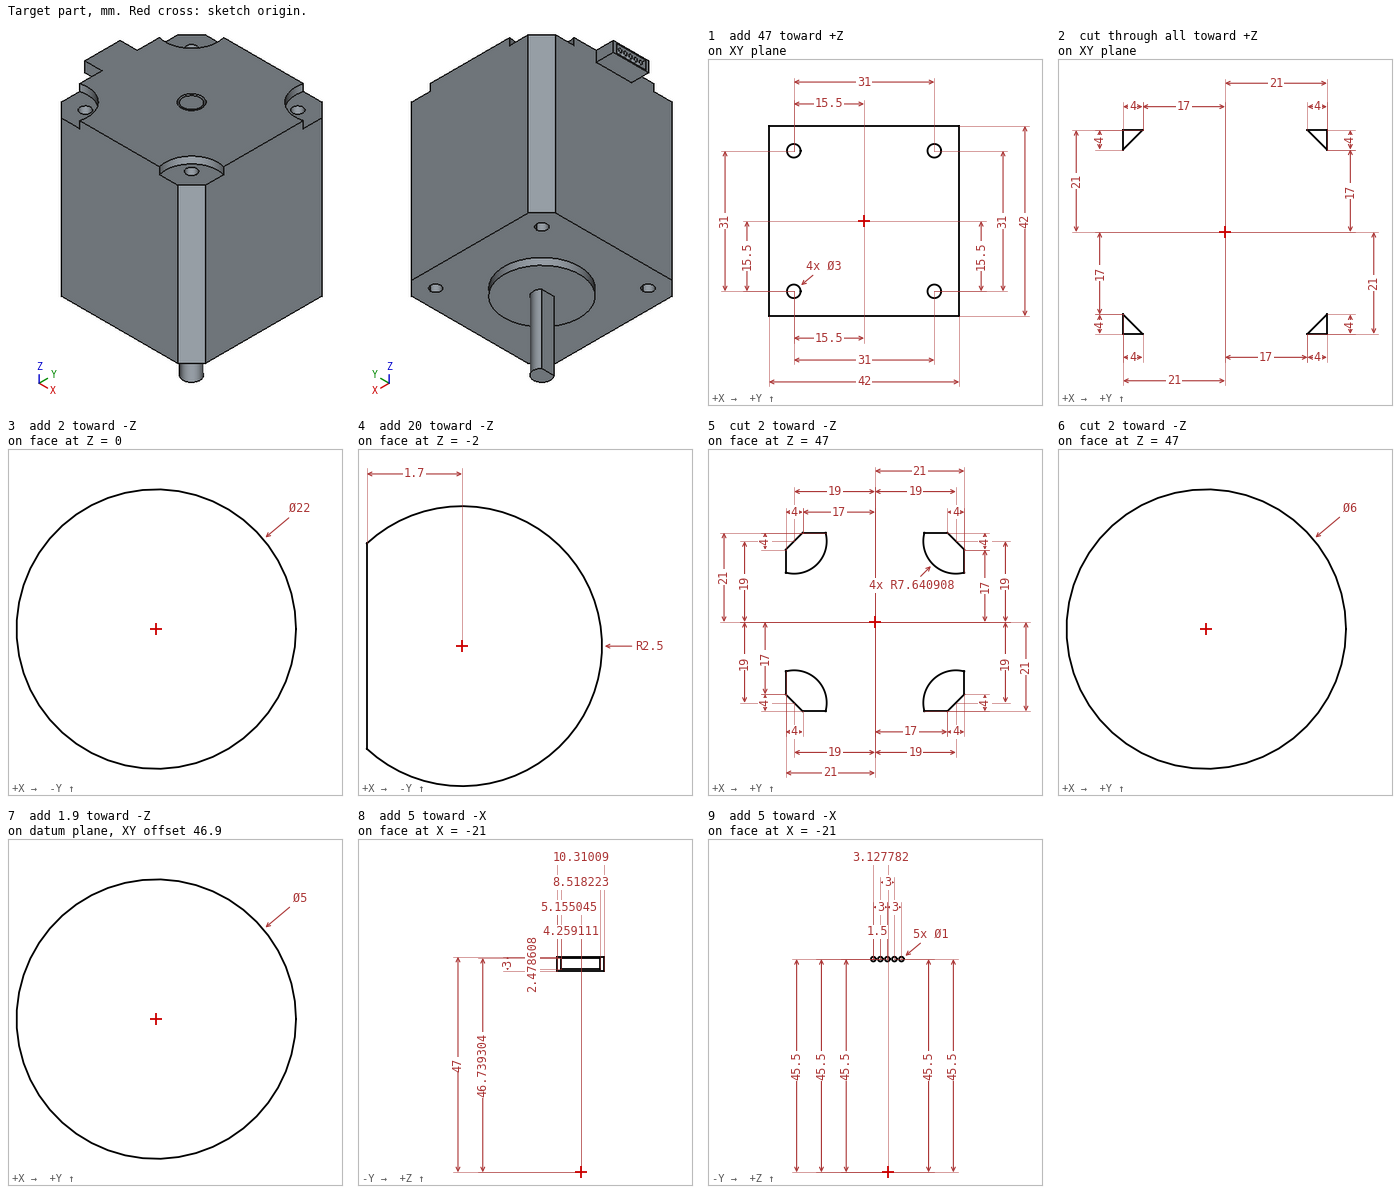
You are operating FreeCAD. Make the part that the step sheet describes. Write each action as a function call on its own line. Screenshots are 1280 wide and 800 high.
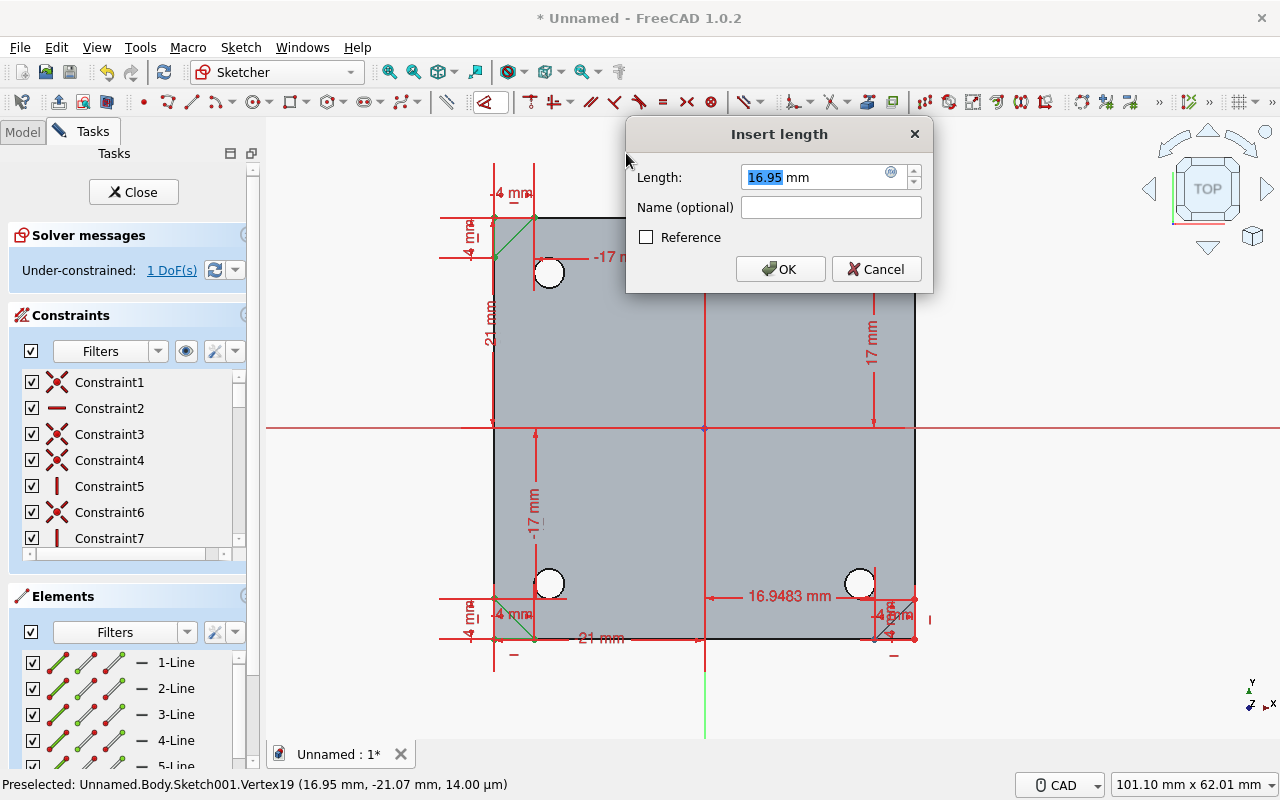
text(17)
key(Return)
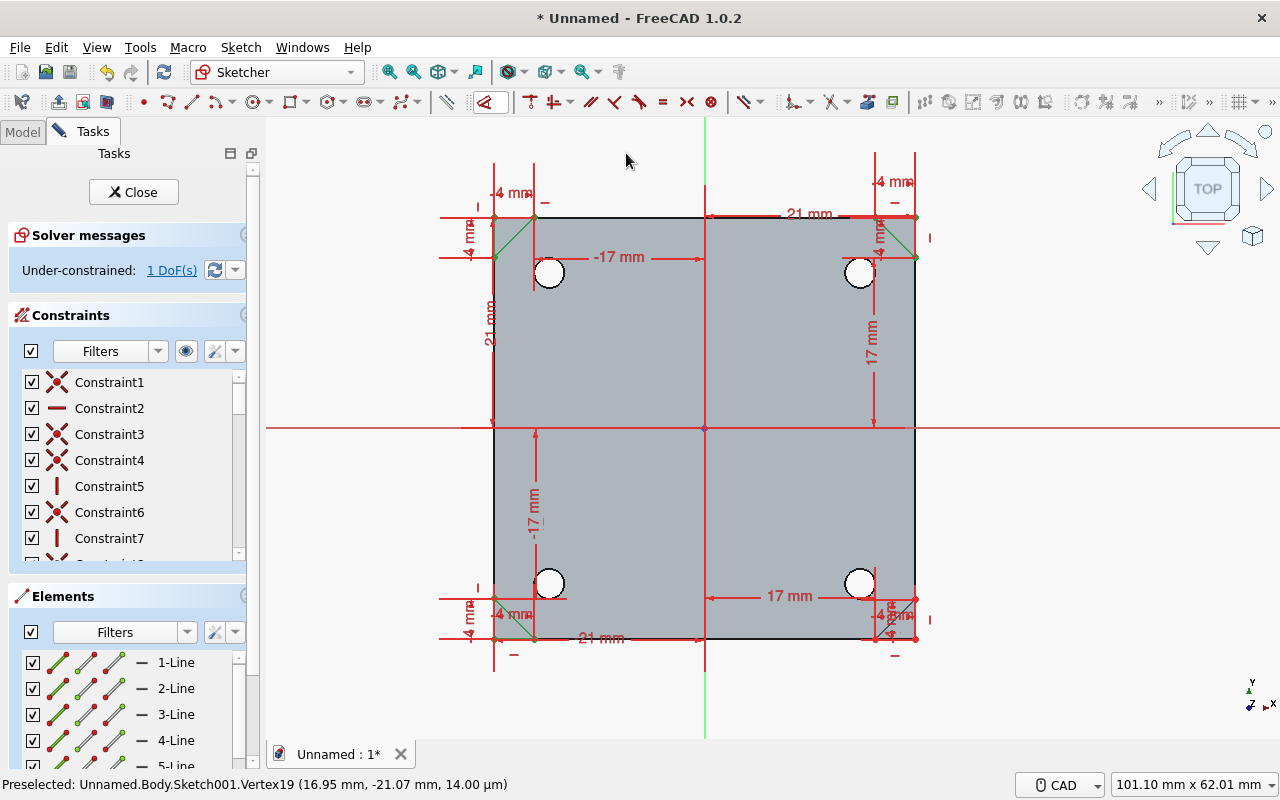
click(875, 640)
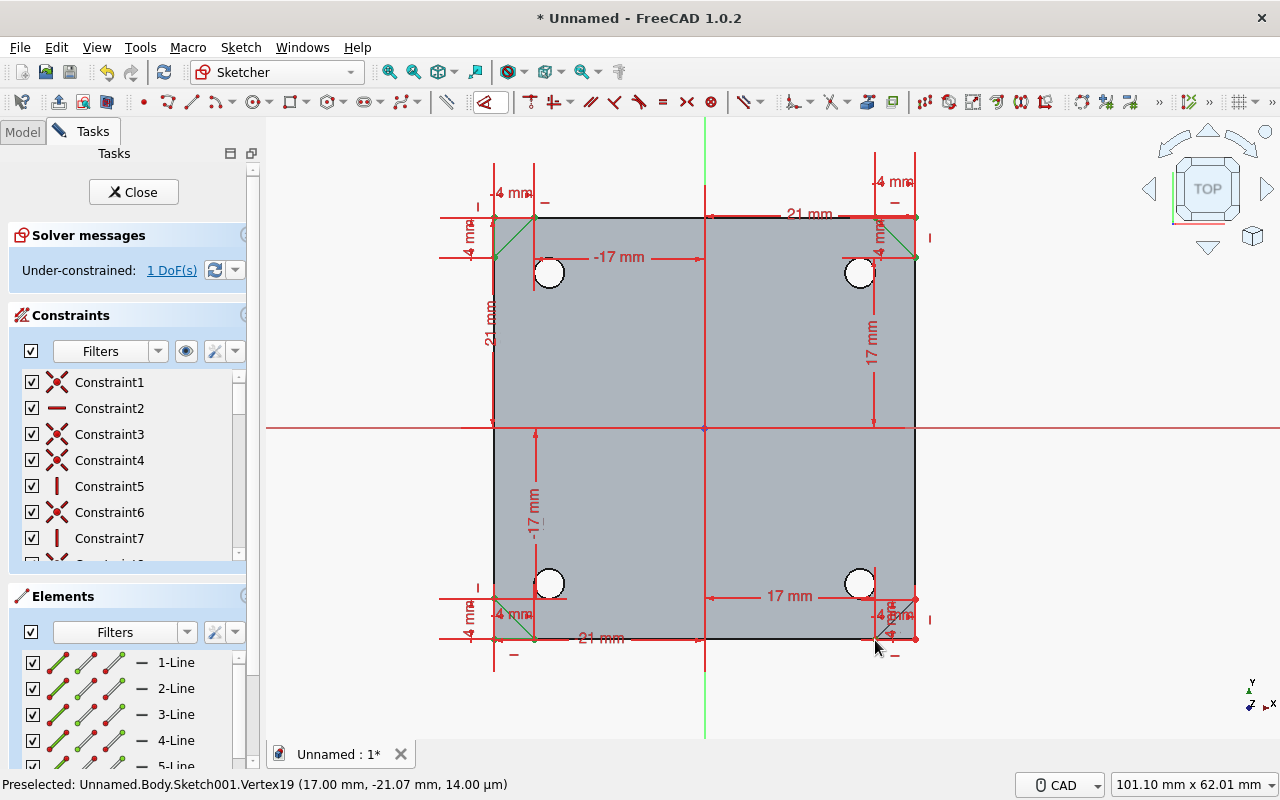
key(i)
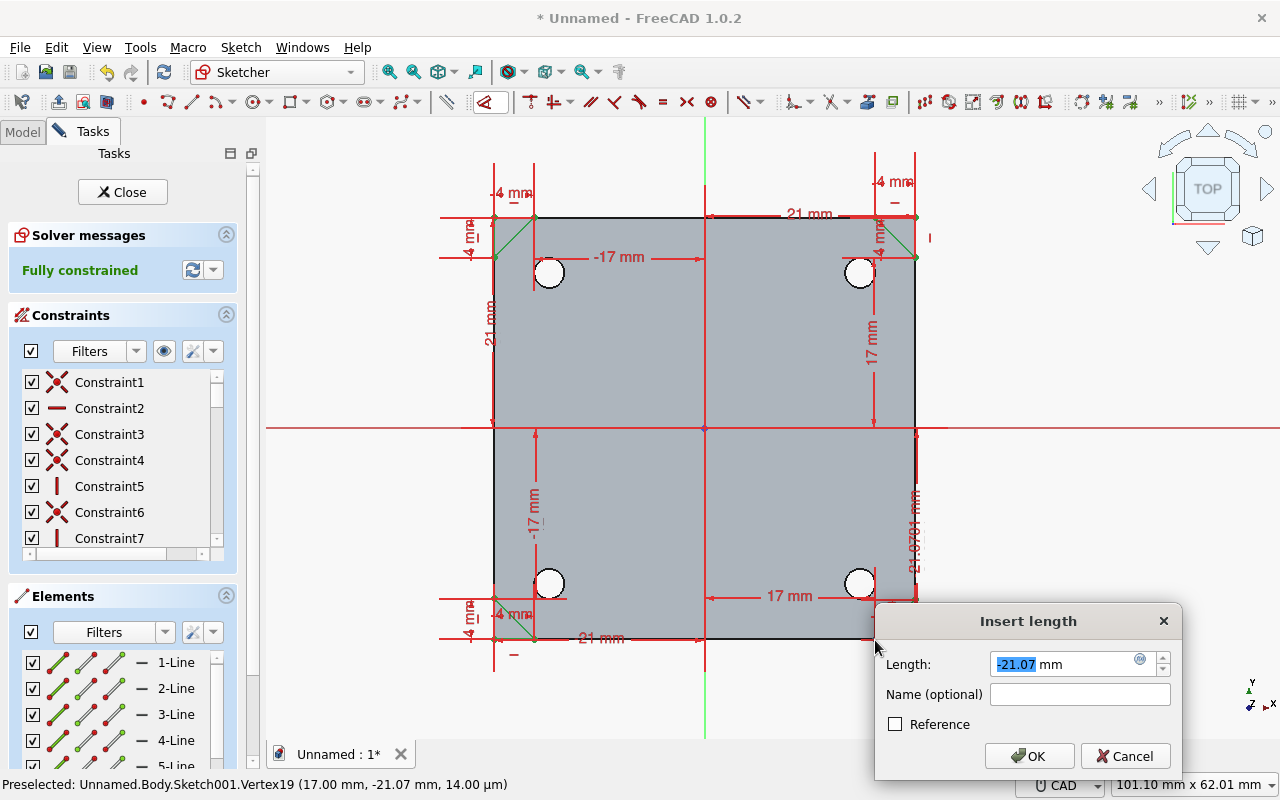
text(-21)
key(Return)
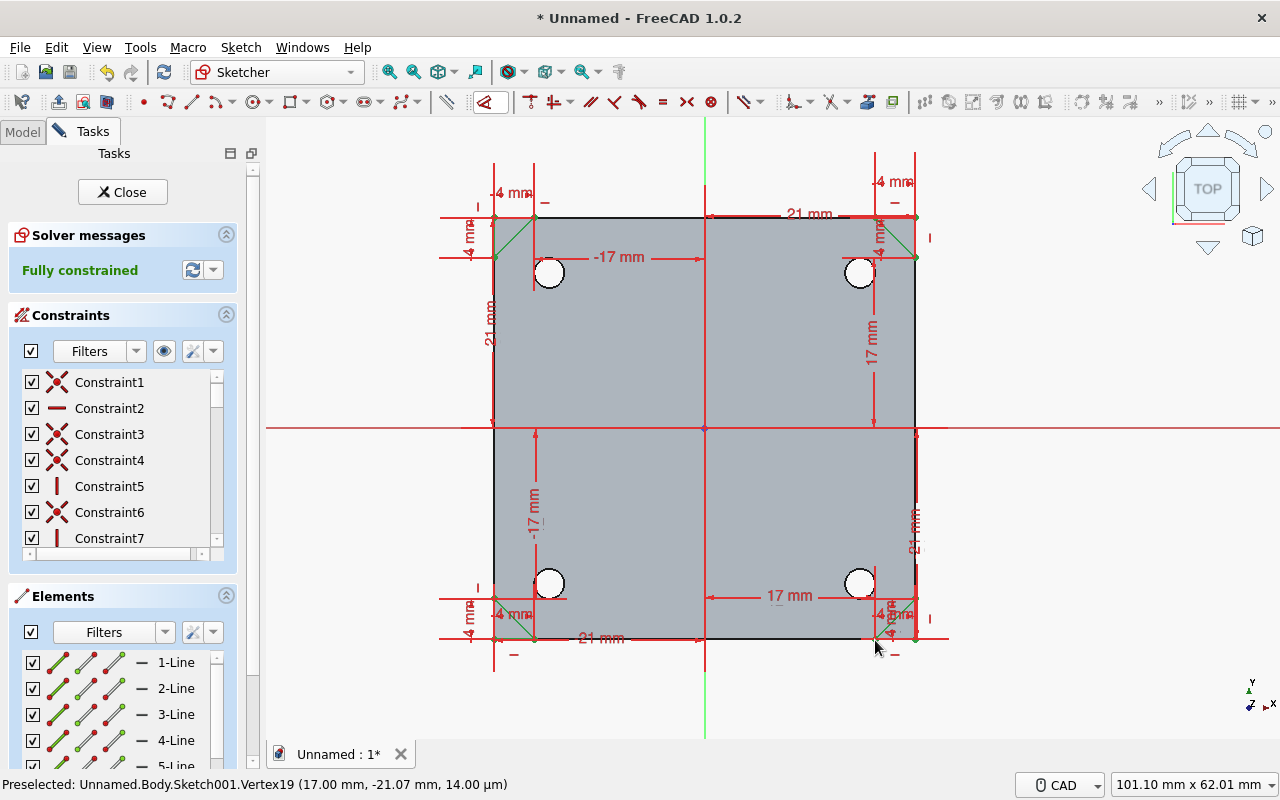
click(123, 192)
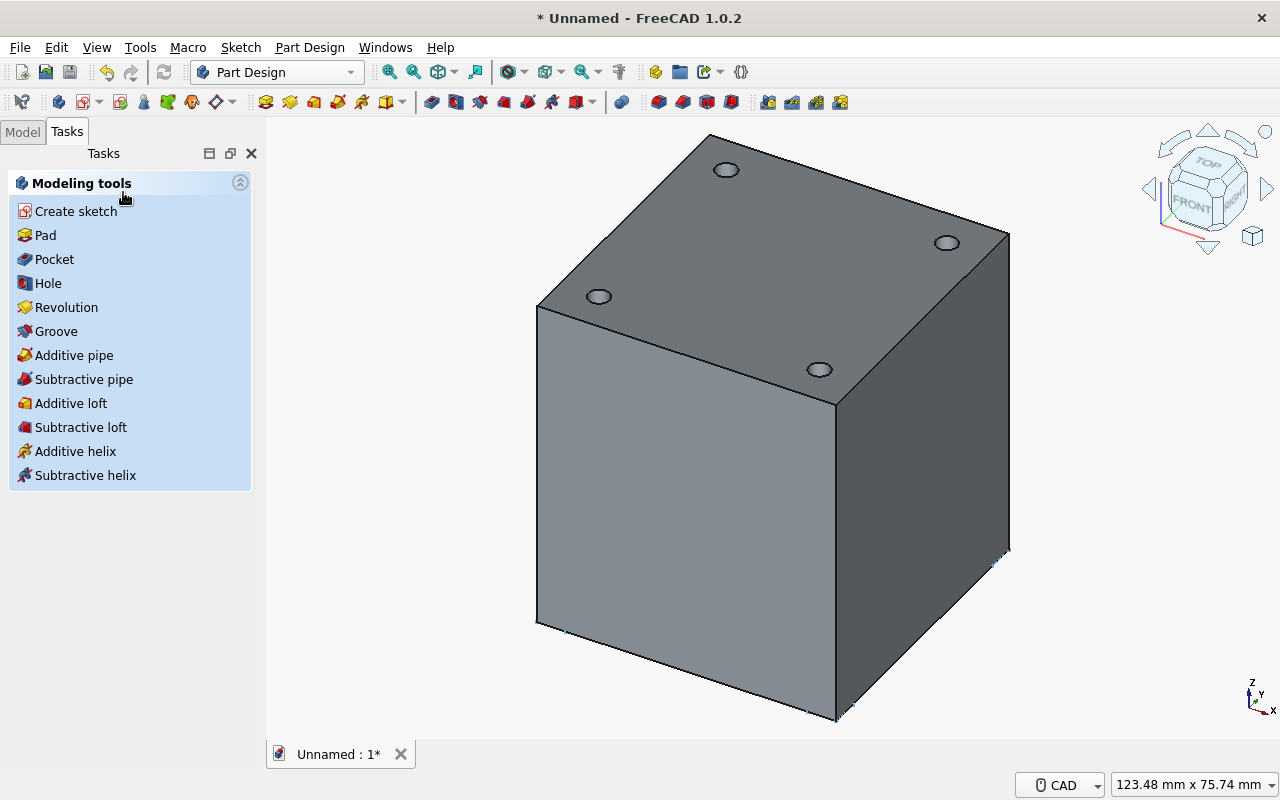
click(432, 102)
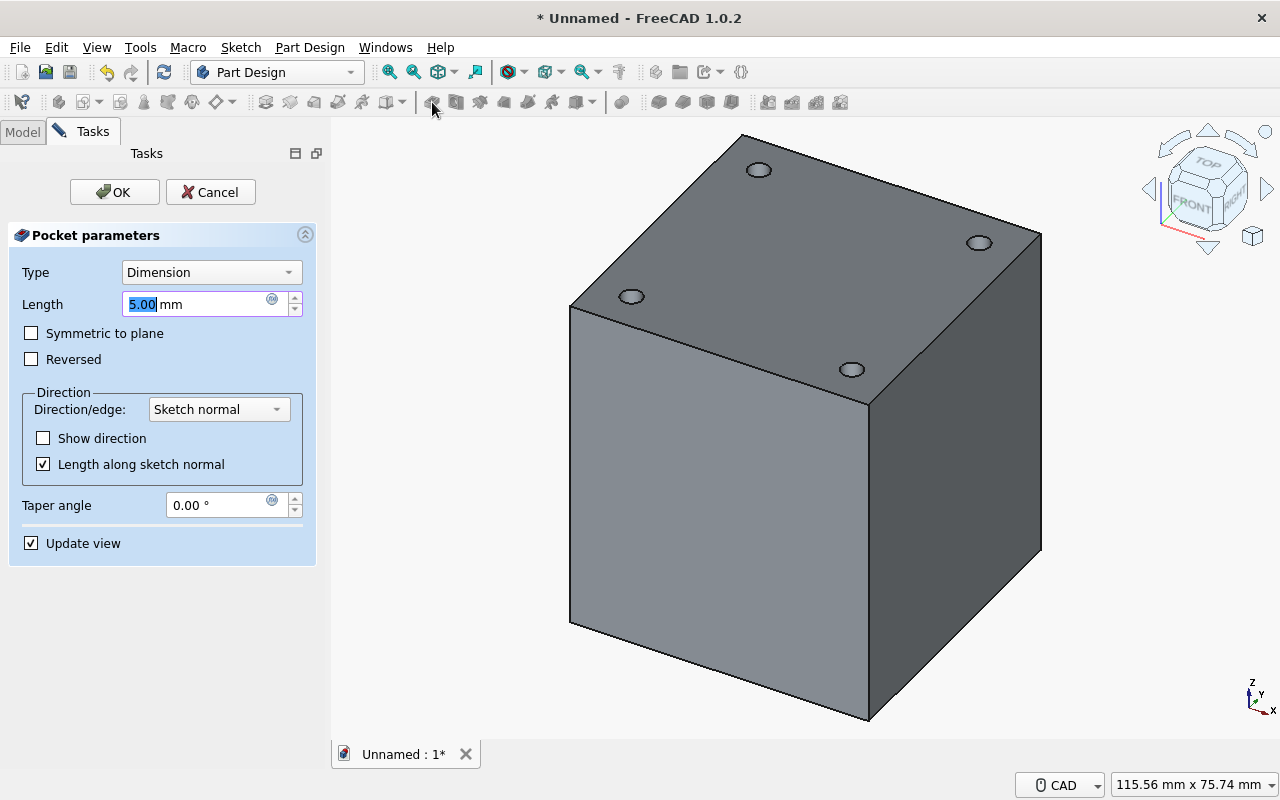
click(212, 272)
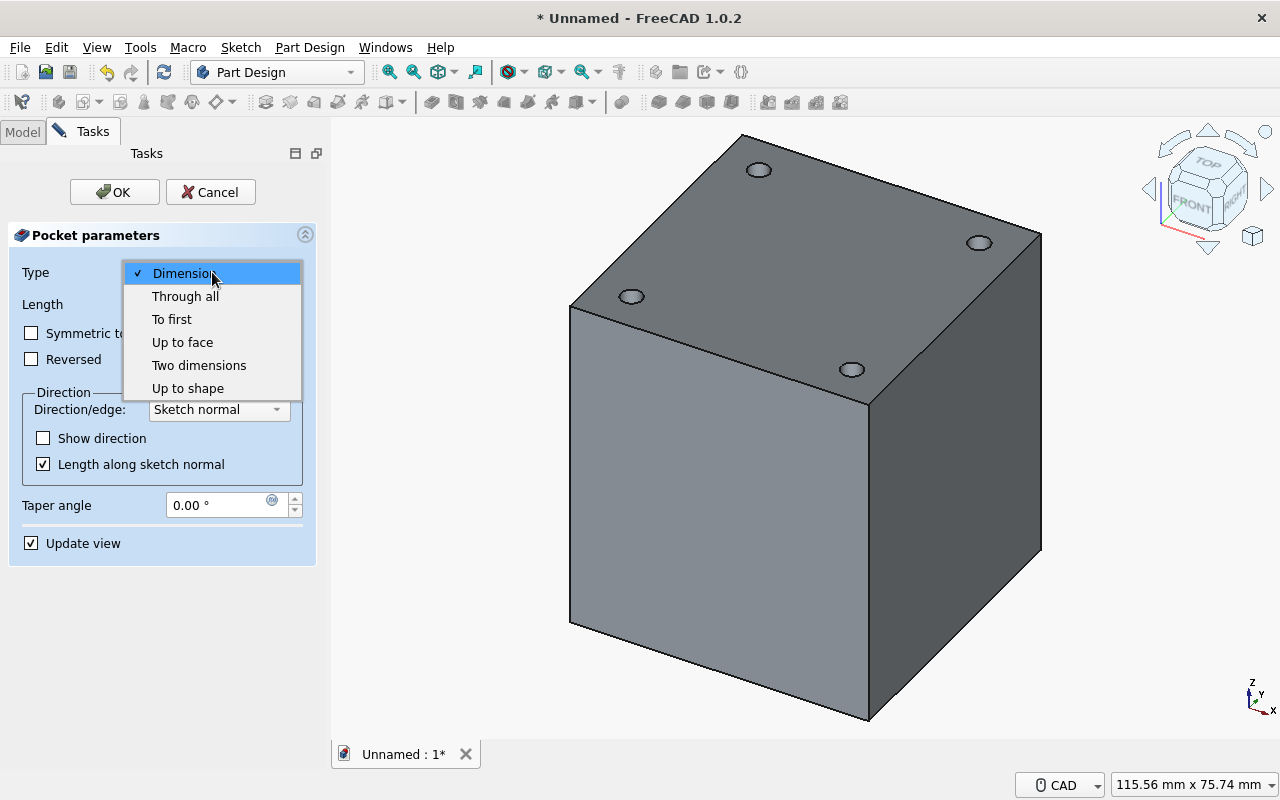
click(212, 296)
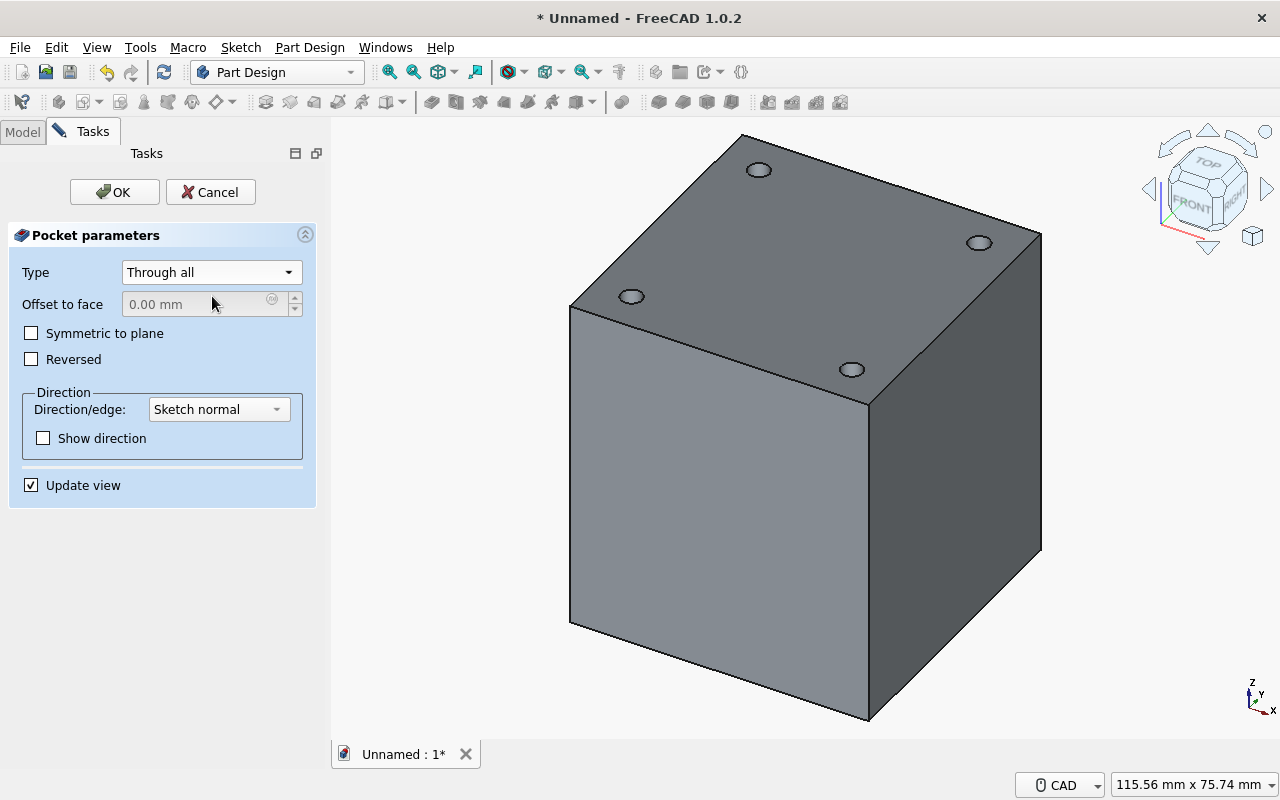
click(30, 359)